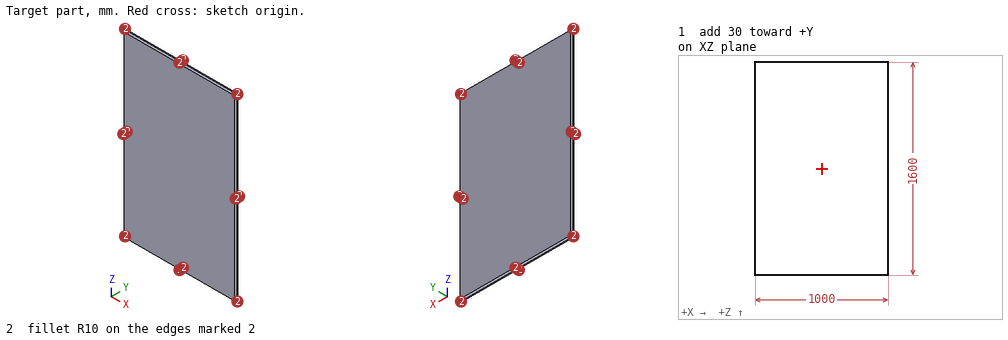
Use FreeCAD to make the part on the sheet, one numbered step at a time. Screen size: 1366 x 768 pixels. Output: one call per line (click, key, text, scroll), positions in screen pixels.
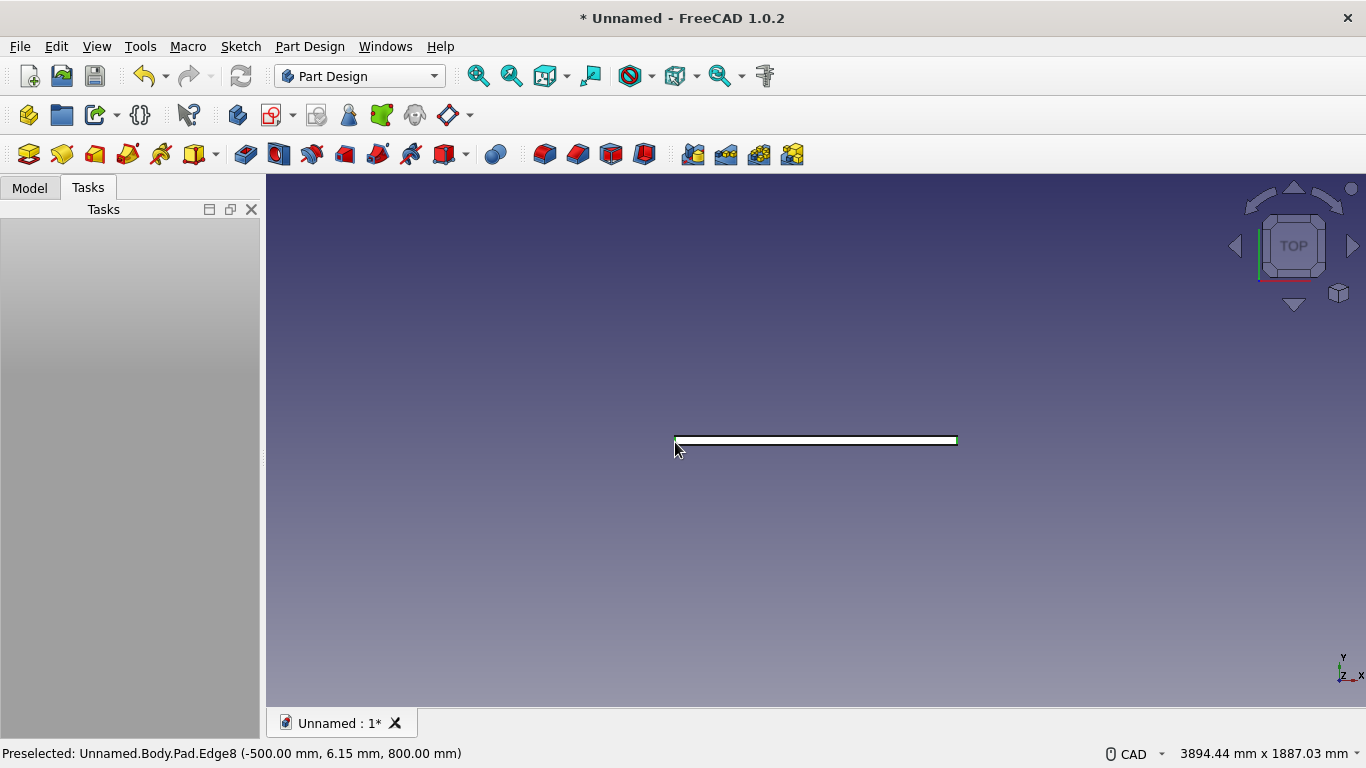
key(1)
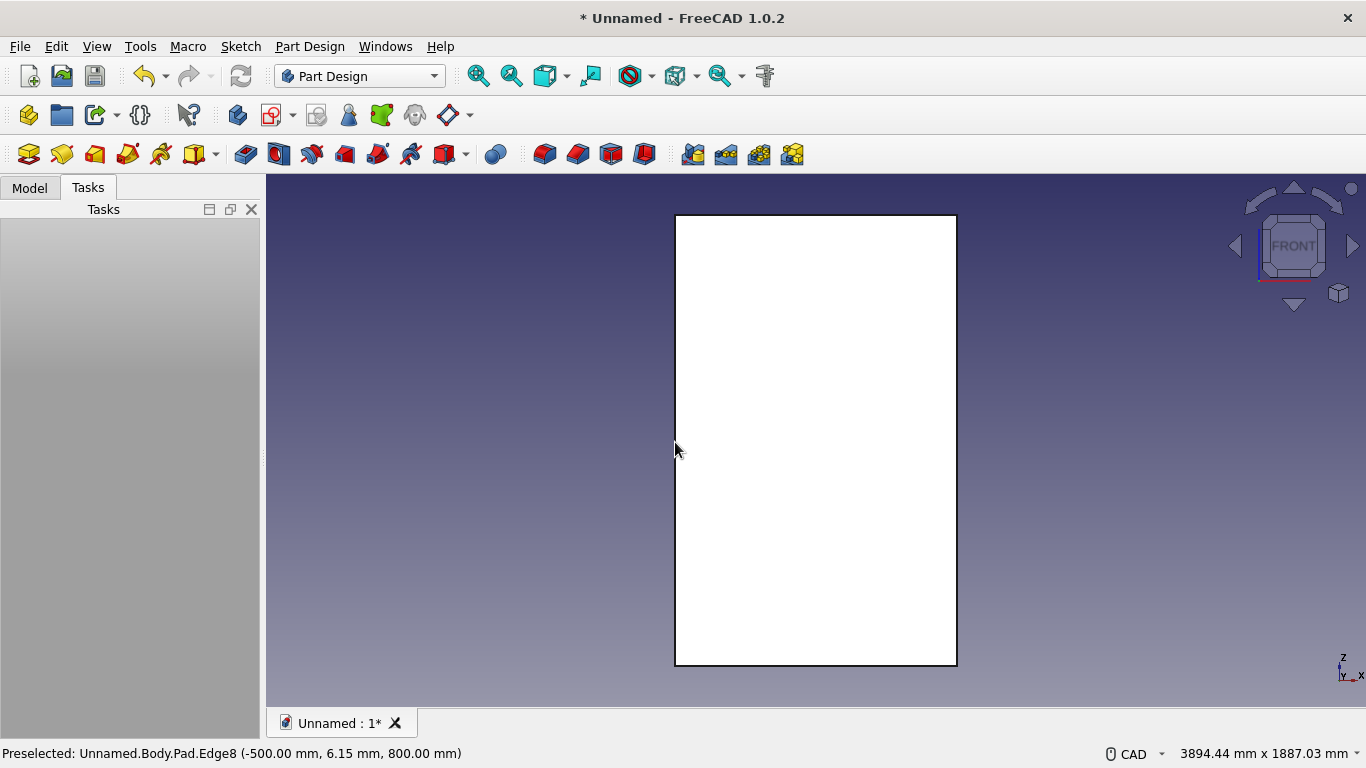
key(3)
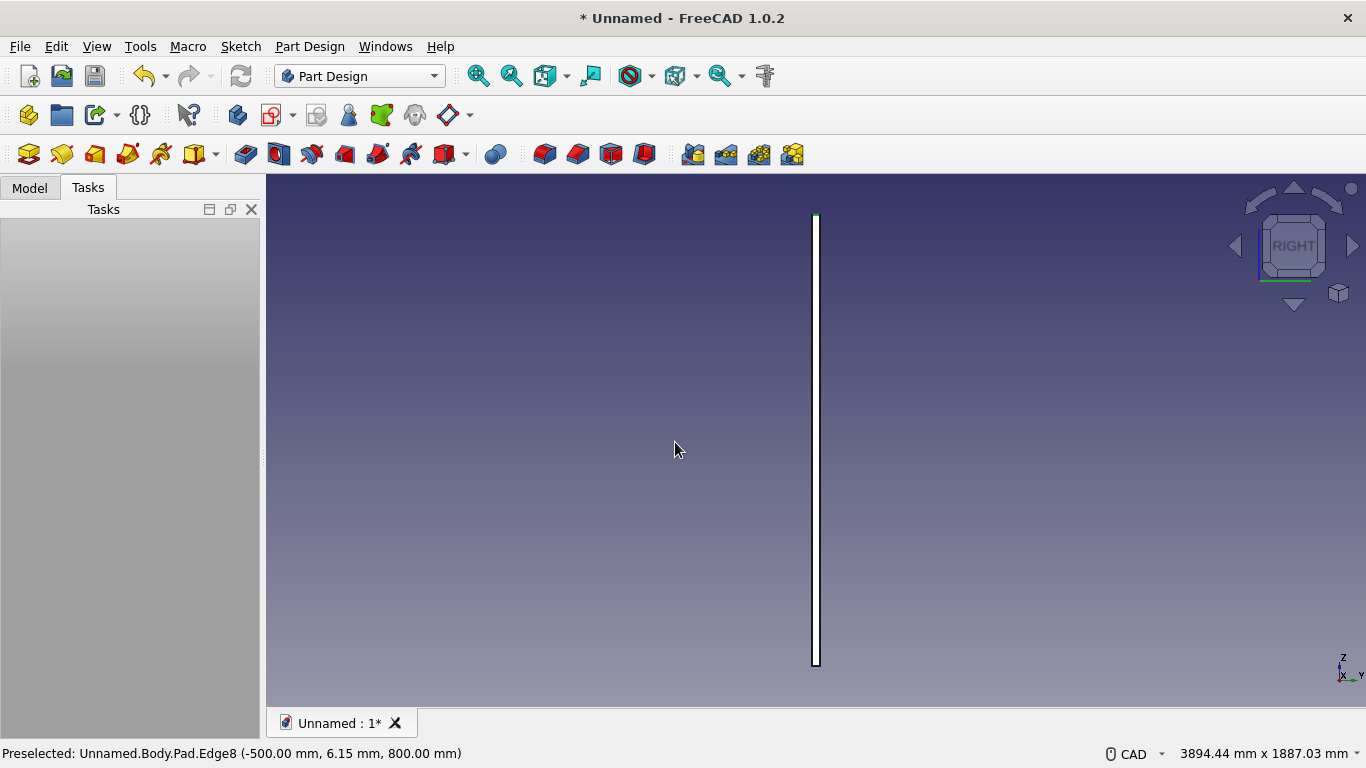
key(5)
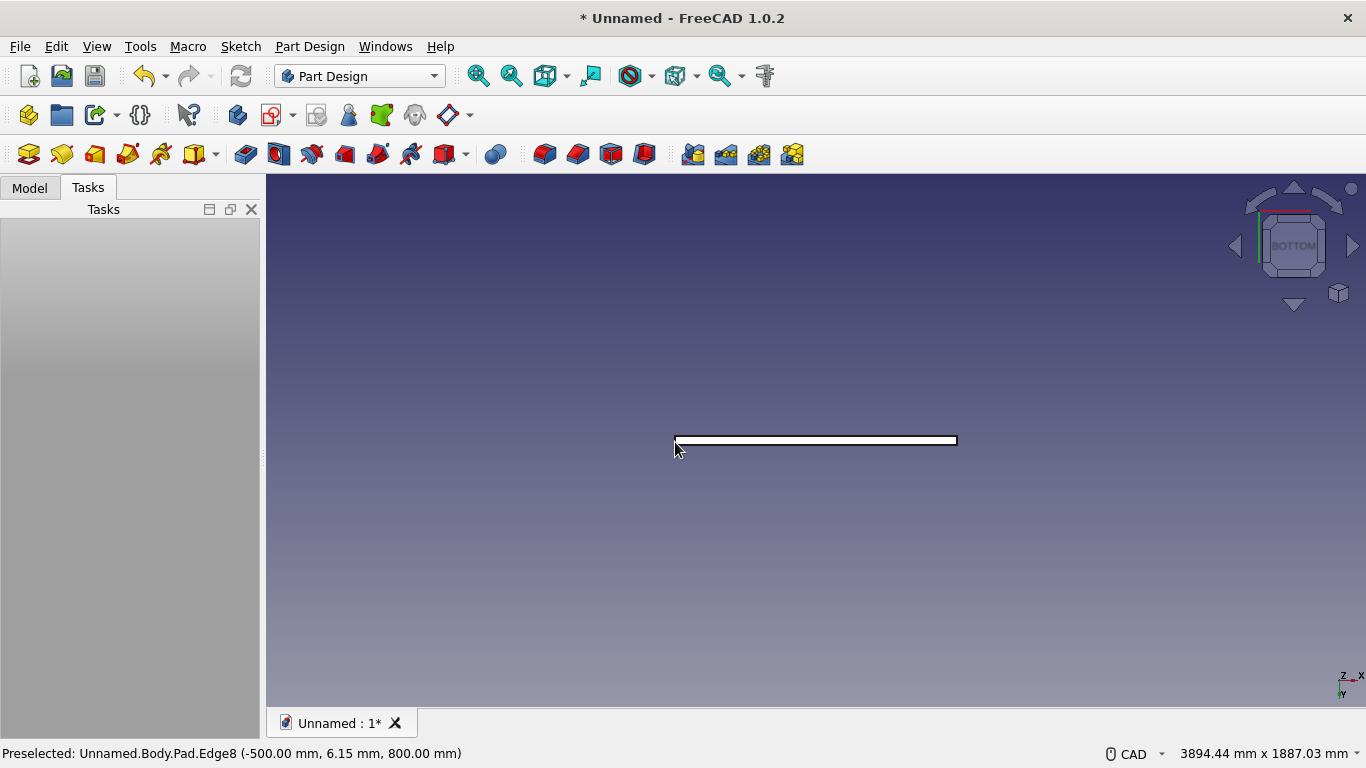
key(v)
key(f)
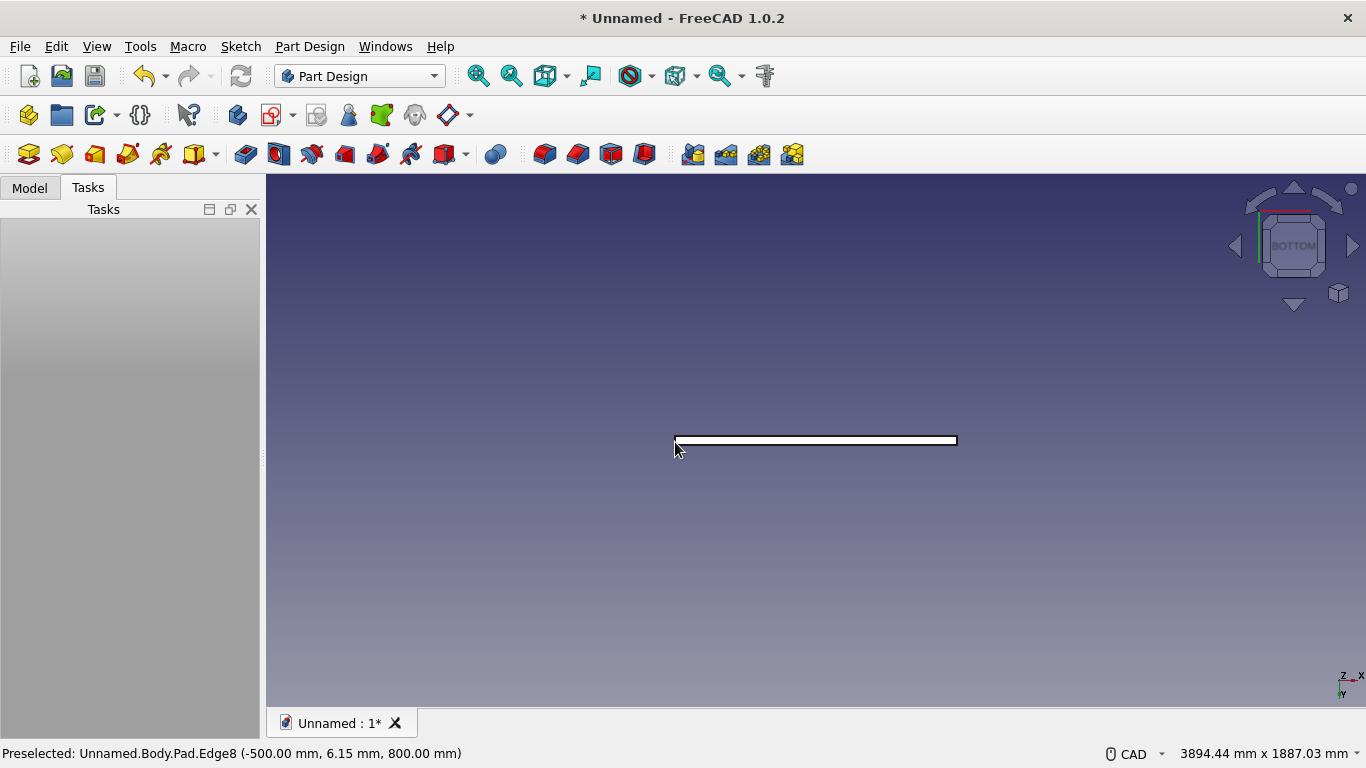
click(675, 442, ctrl)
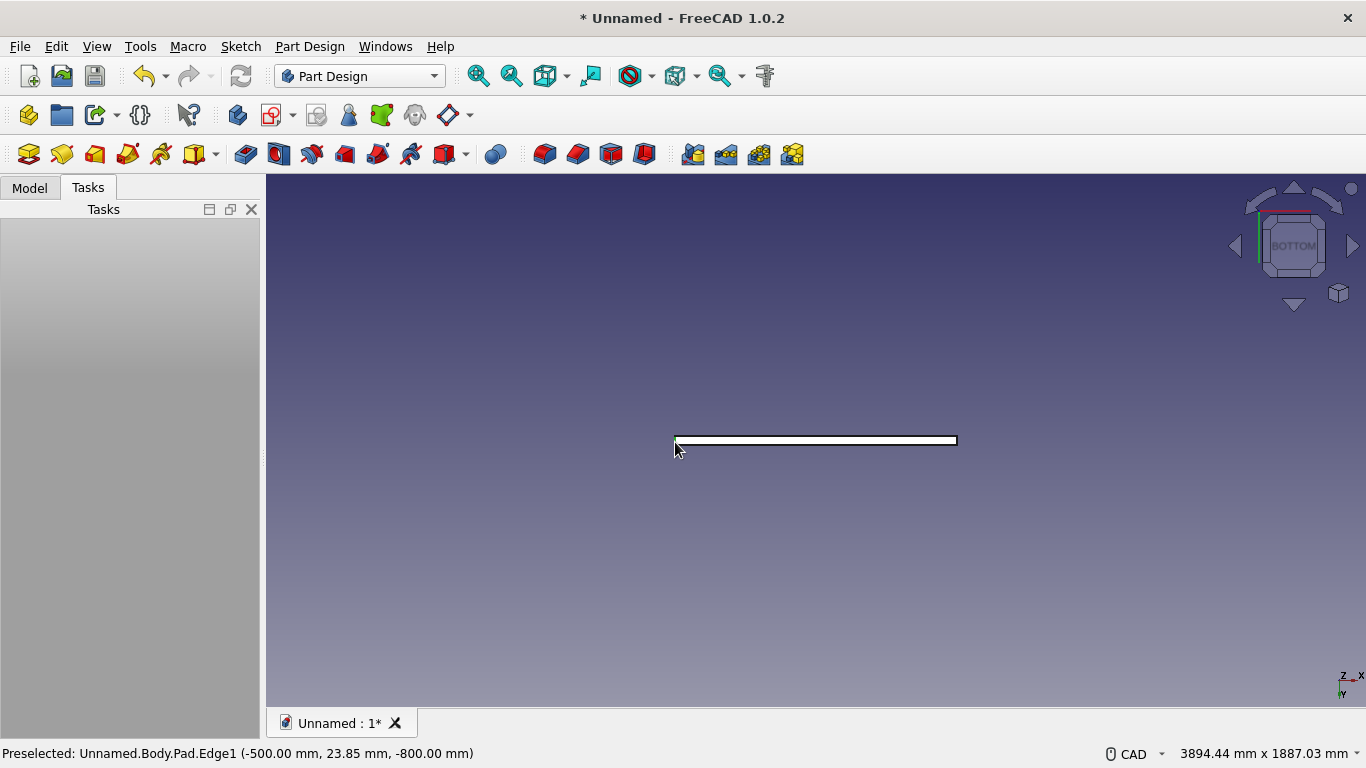
click(957, 442, ctrl)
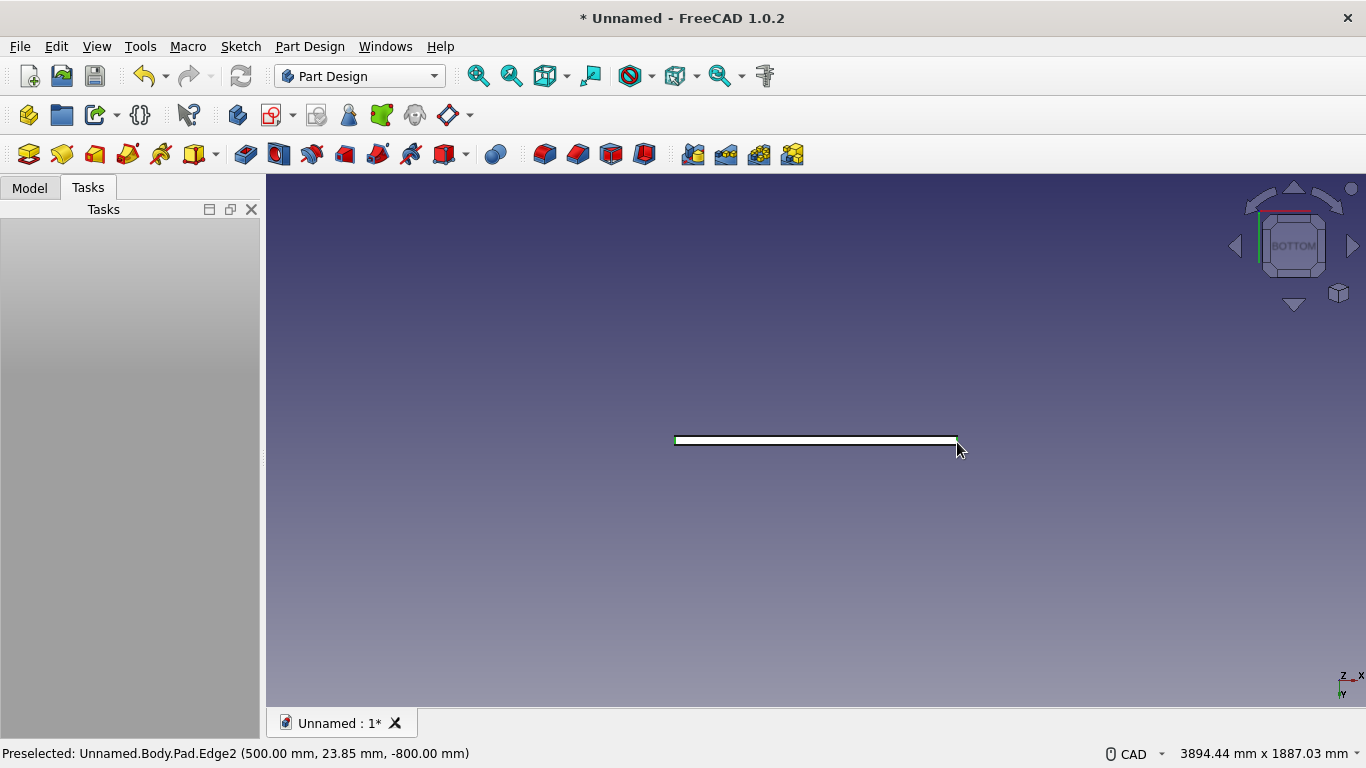
key(4)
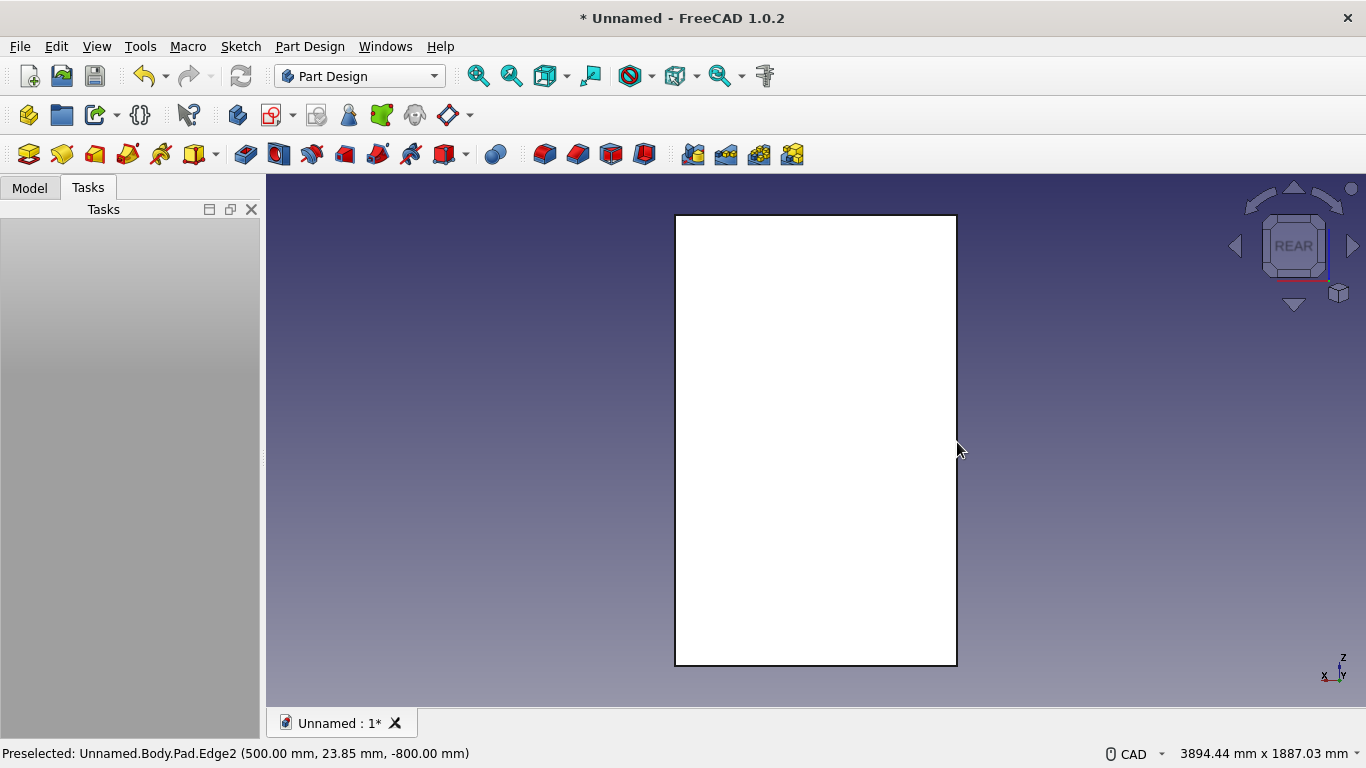
click(816, 375, ctrl)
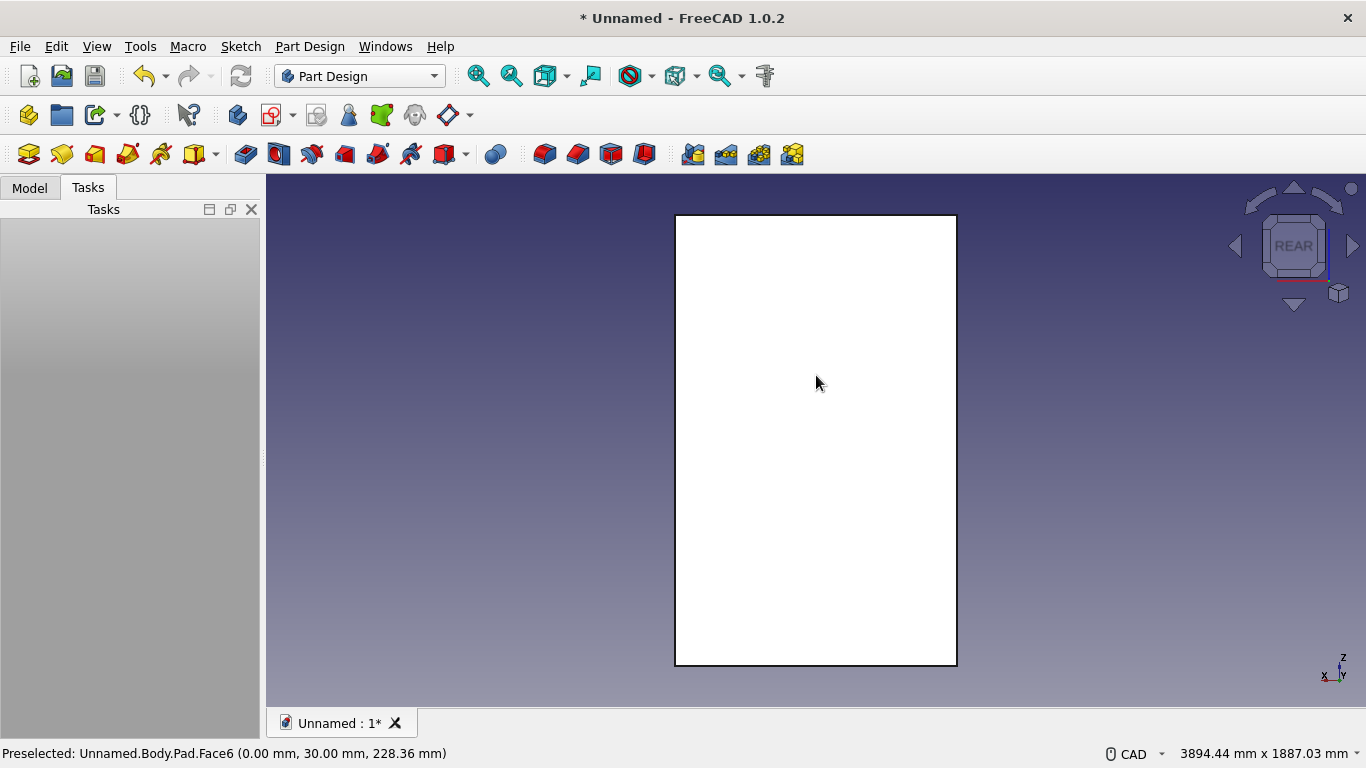
click(545, 154)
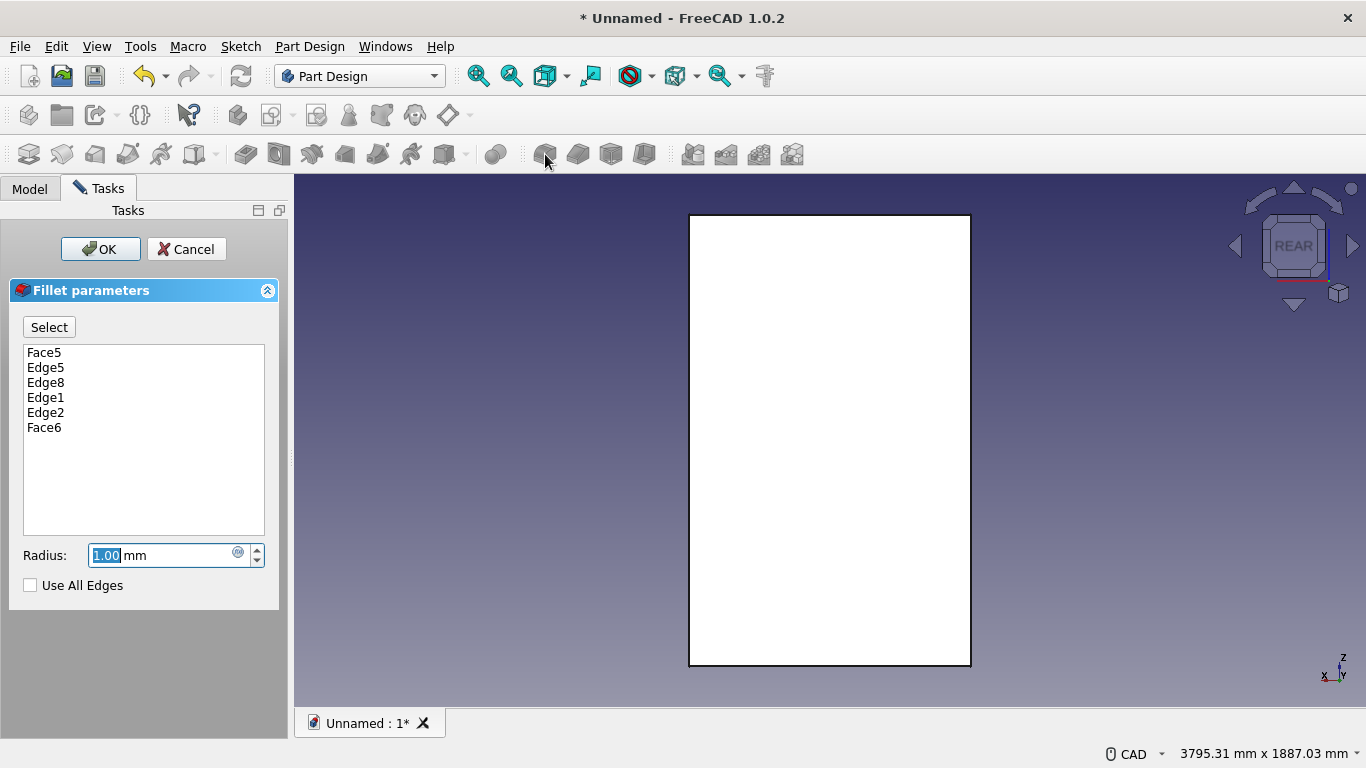
text(10)
key(Tab)